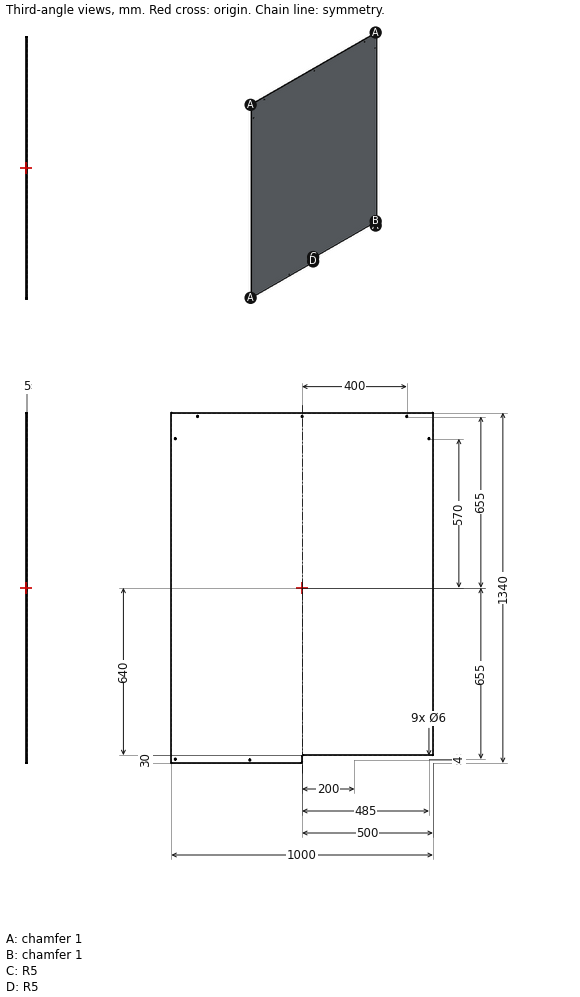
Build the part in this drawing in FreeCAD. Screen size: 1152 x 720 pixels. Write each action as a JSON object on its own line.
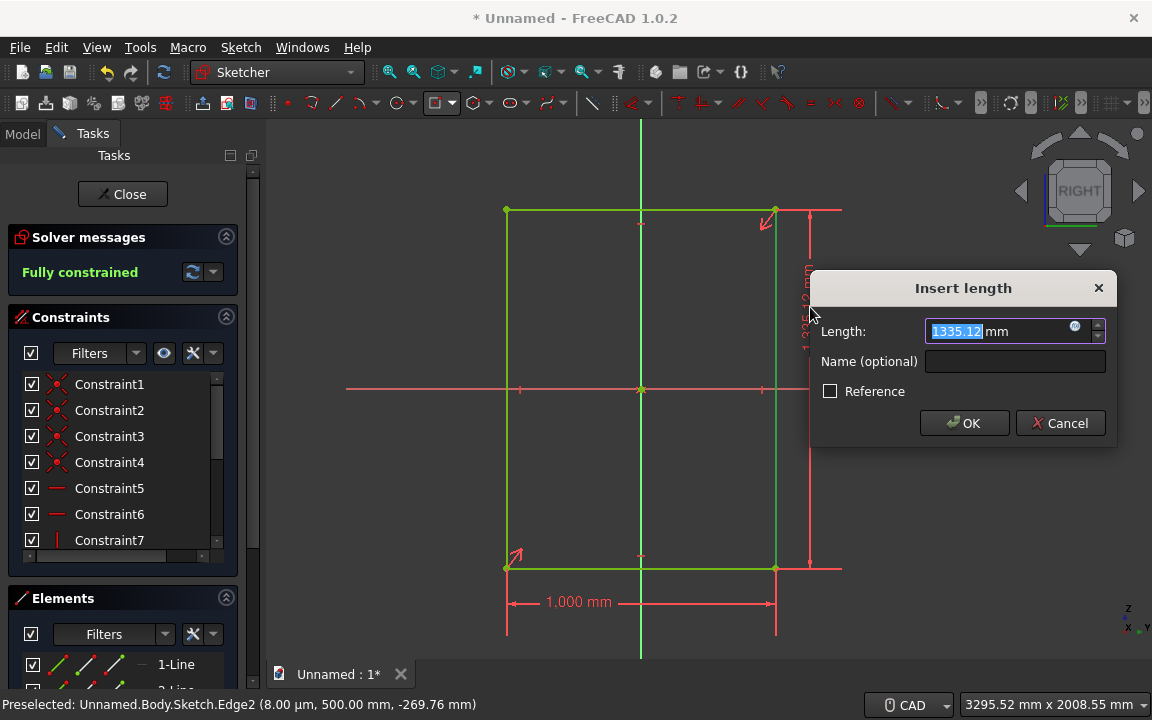
{"action": "type", "text": "1340"}
{"action": "key", "text": "Return"}
{"action": "key", "text": "Escape"}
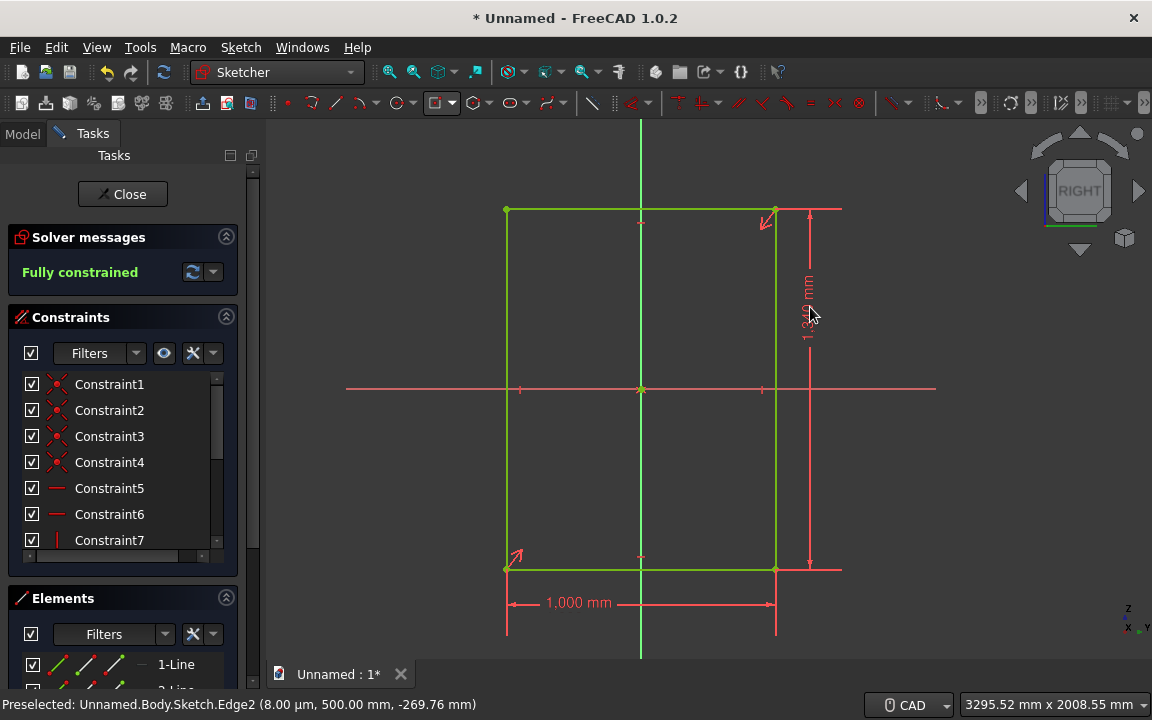
{"action": "left_click", "coordinate": [123, 194]}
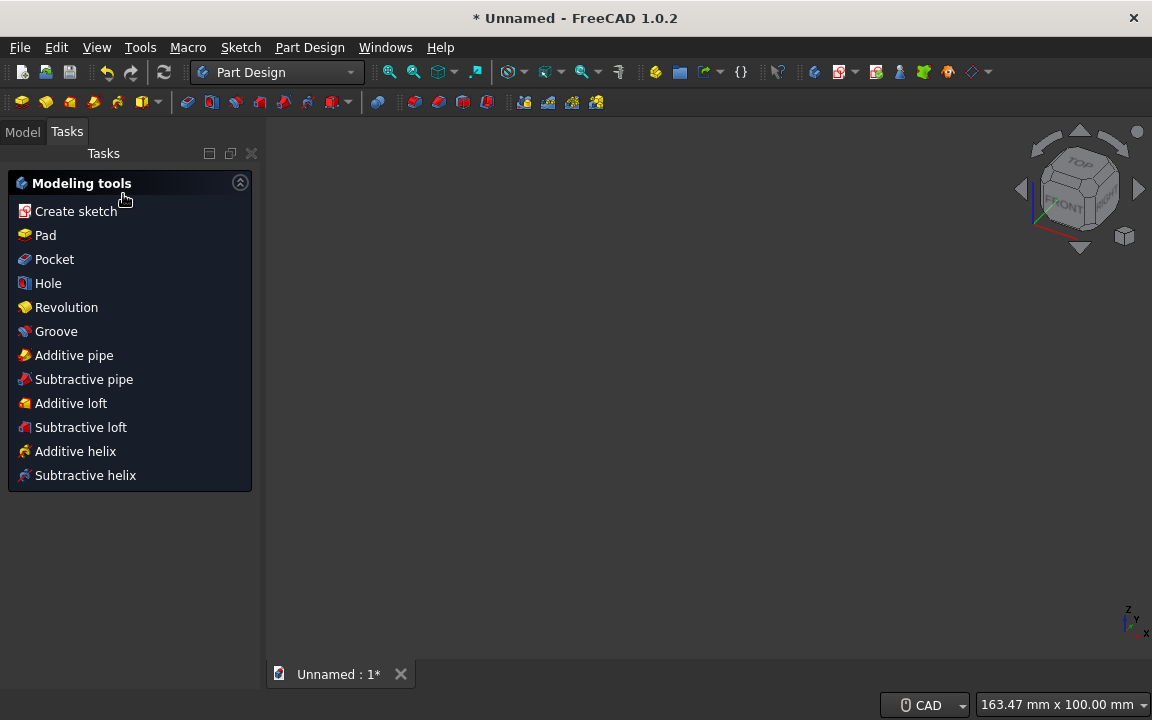
{"action": "left_click", "coordinate": [22, 102]}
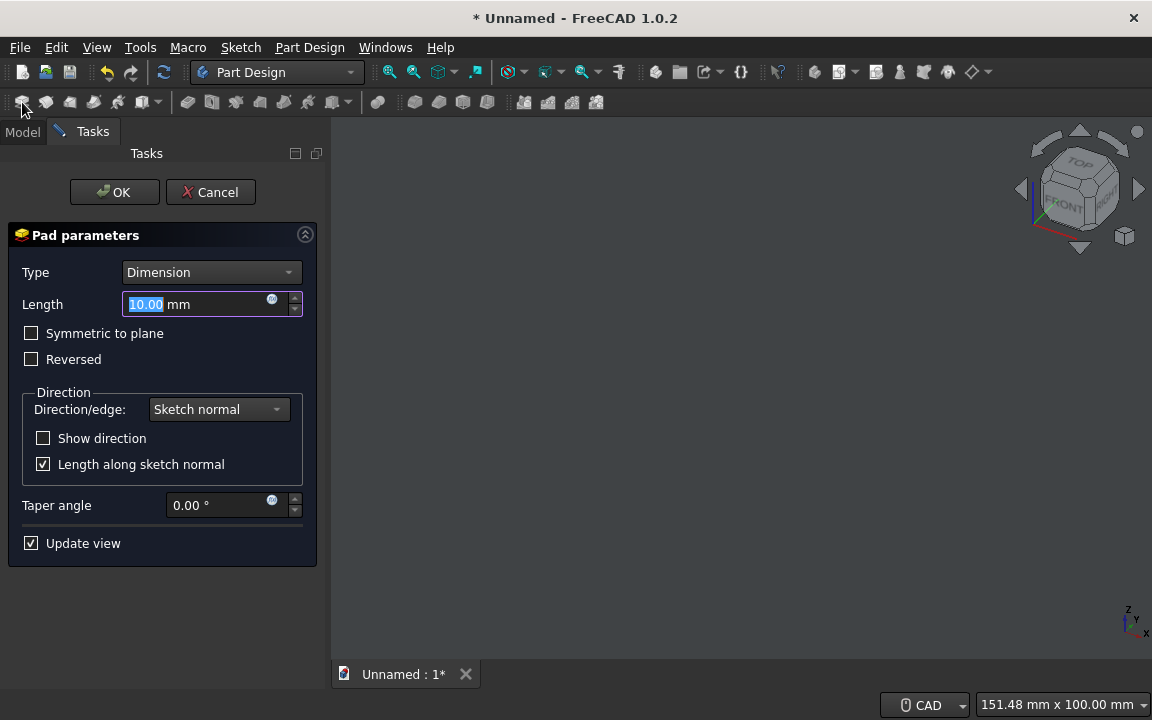
{"action": "type", "text": "5"}
{"action": "key", "text": "Tab"}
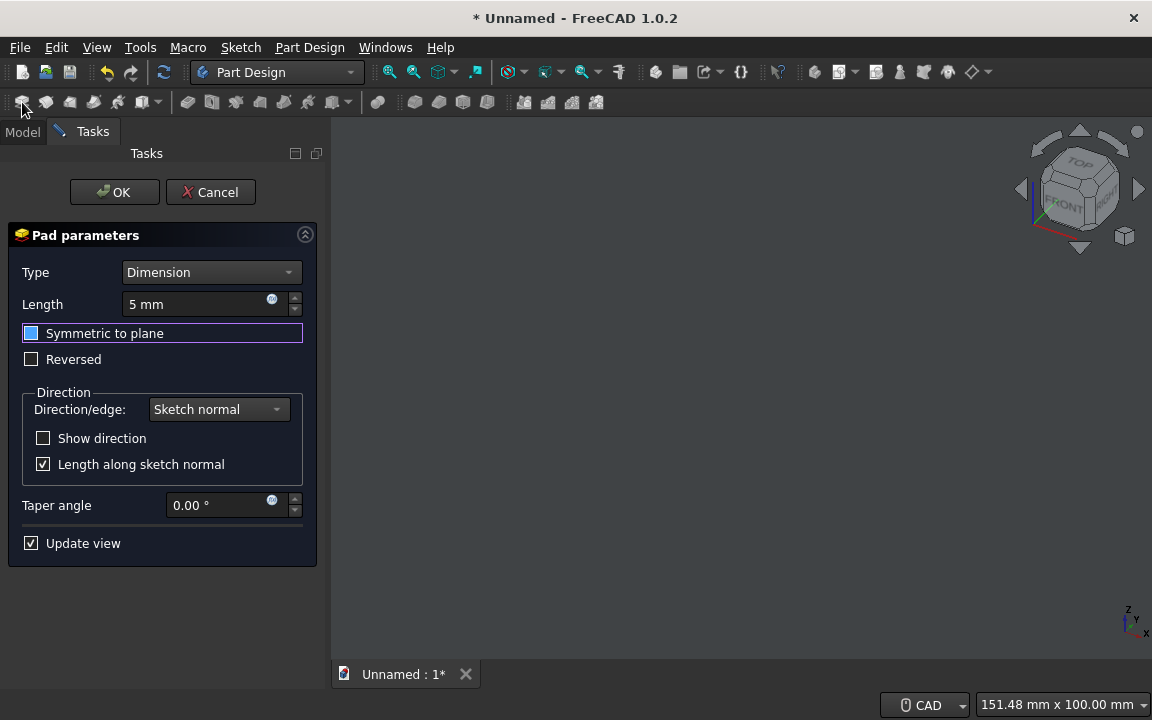
{"action": "left_click", "coordinate": [115, 192]}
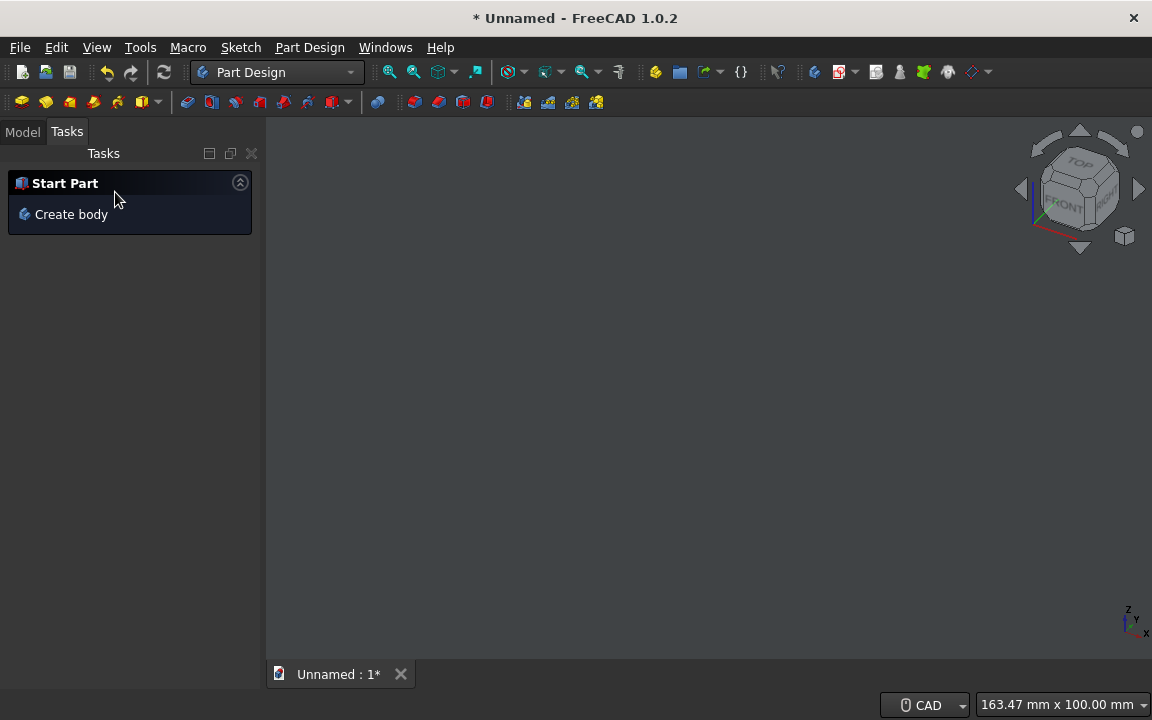
{"action": "left_click", "coordinate": [390, 72]}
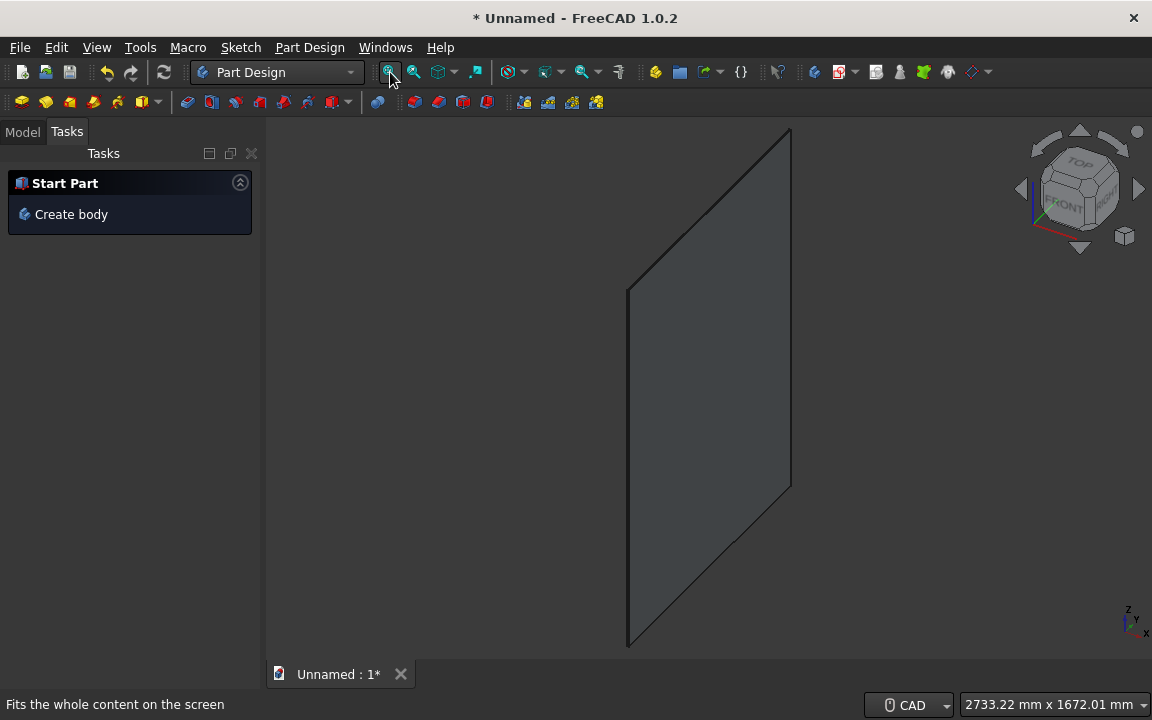
{"action": "key", "text": "0"}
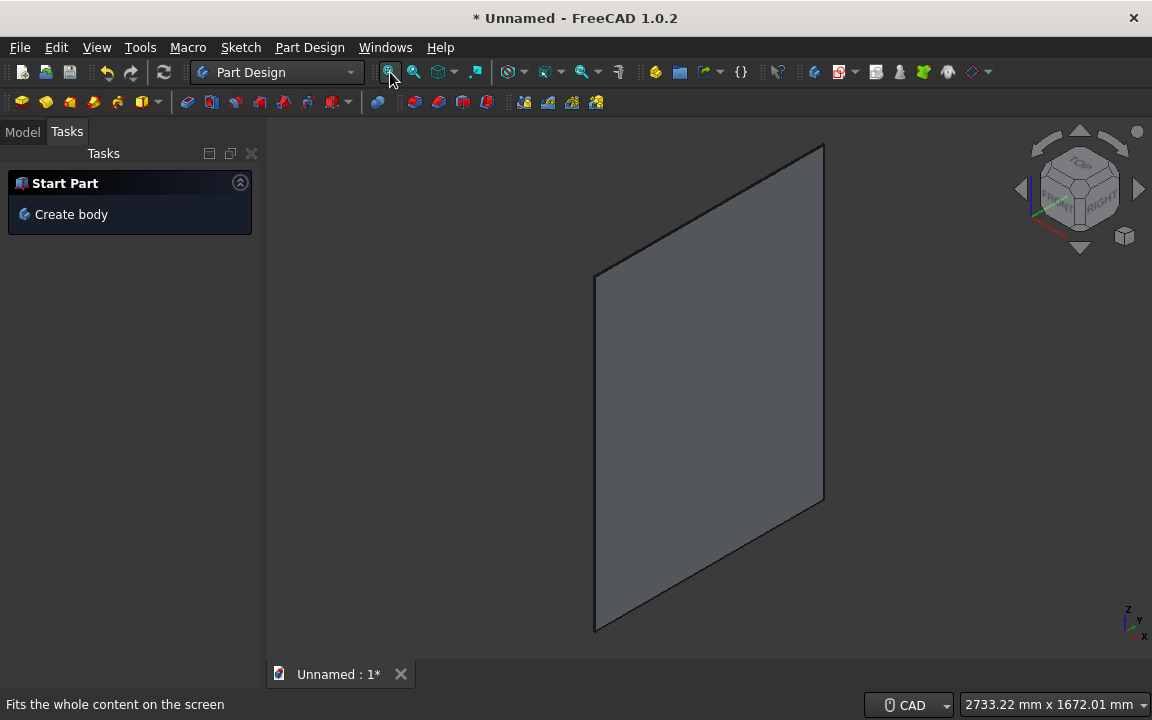
{"action": "key", "text": "2"}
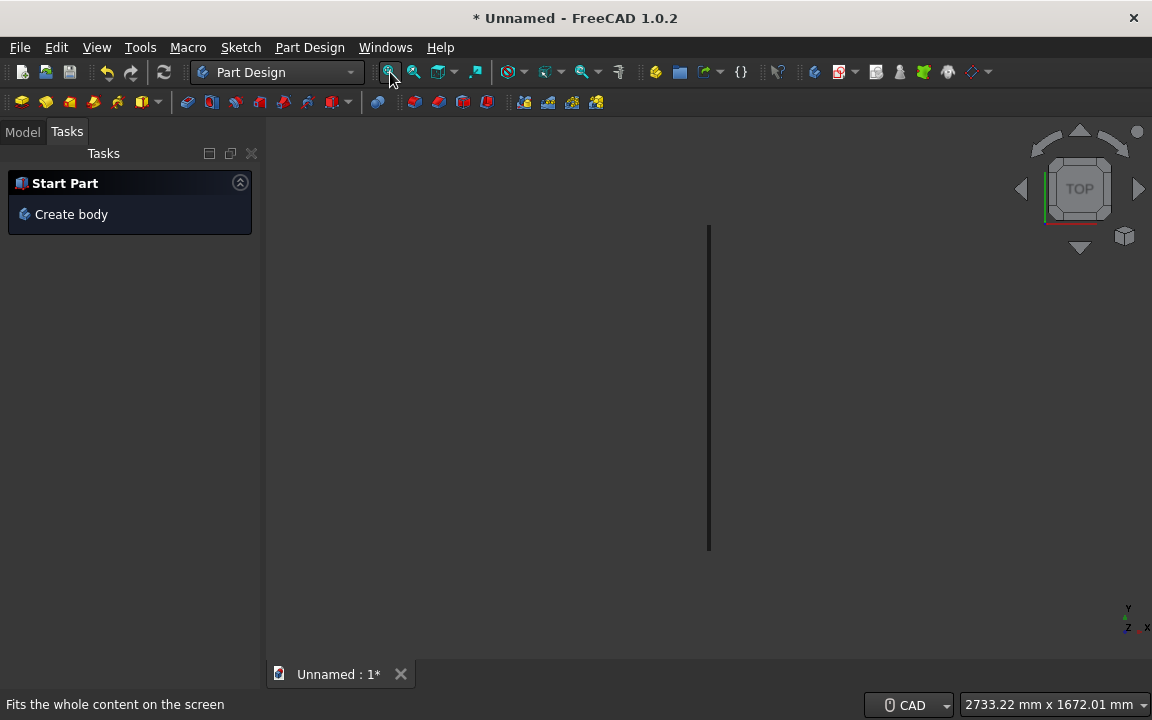
{"action": "scroll", "coordinate": [709, 225], "scroll_direction": "up", "scroll_amount": 15}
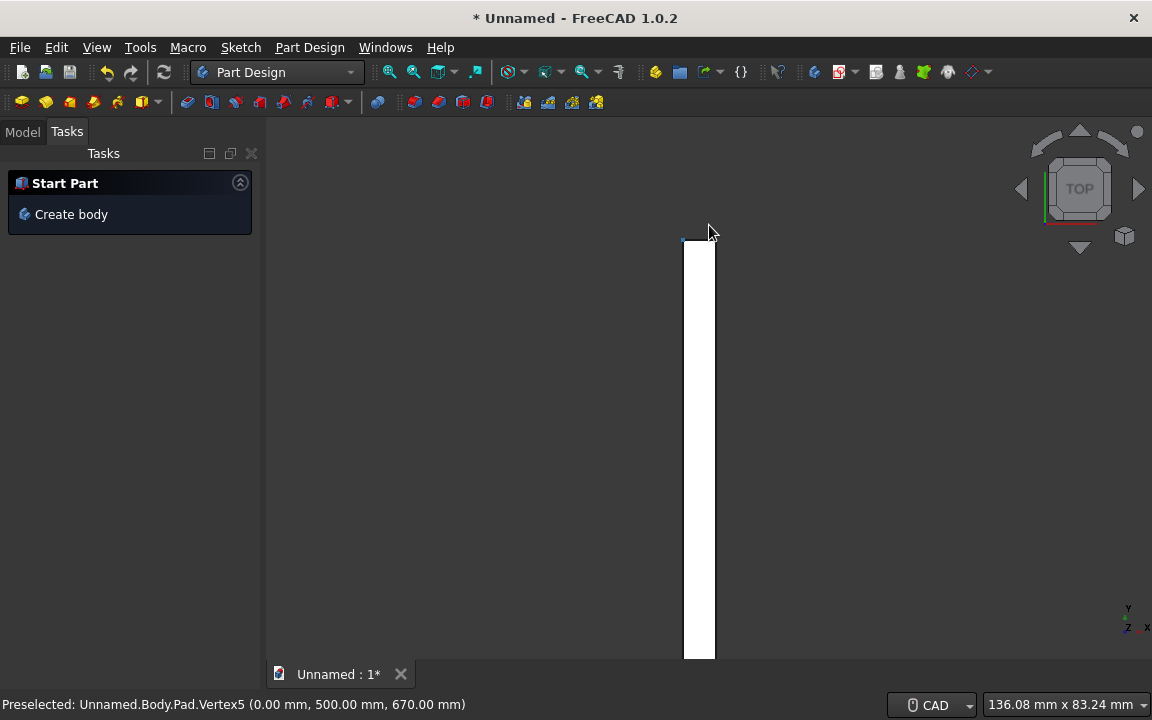
{"action": "left_click", "coordinate": [699, 239]}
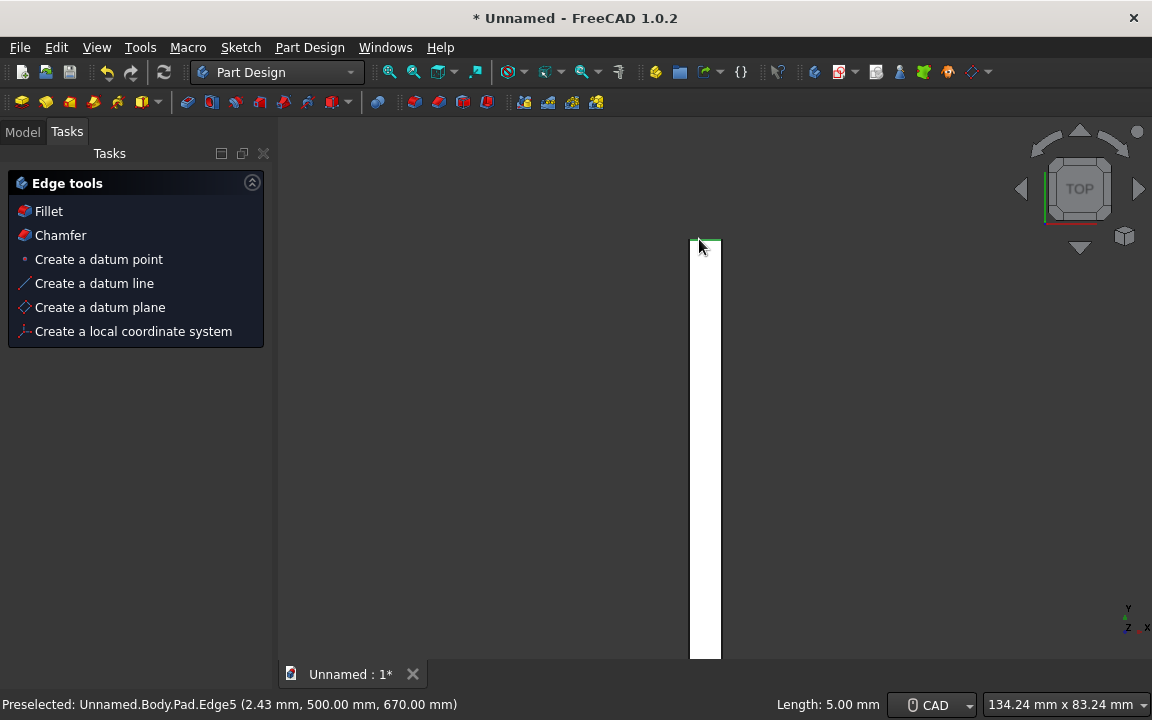
{"action": "left_click", "coordinate": [390, 72]}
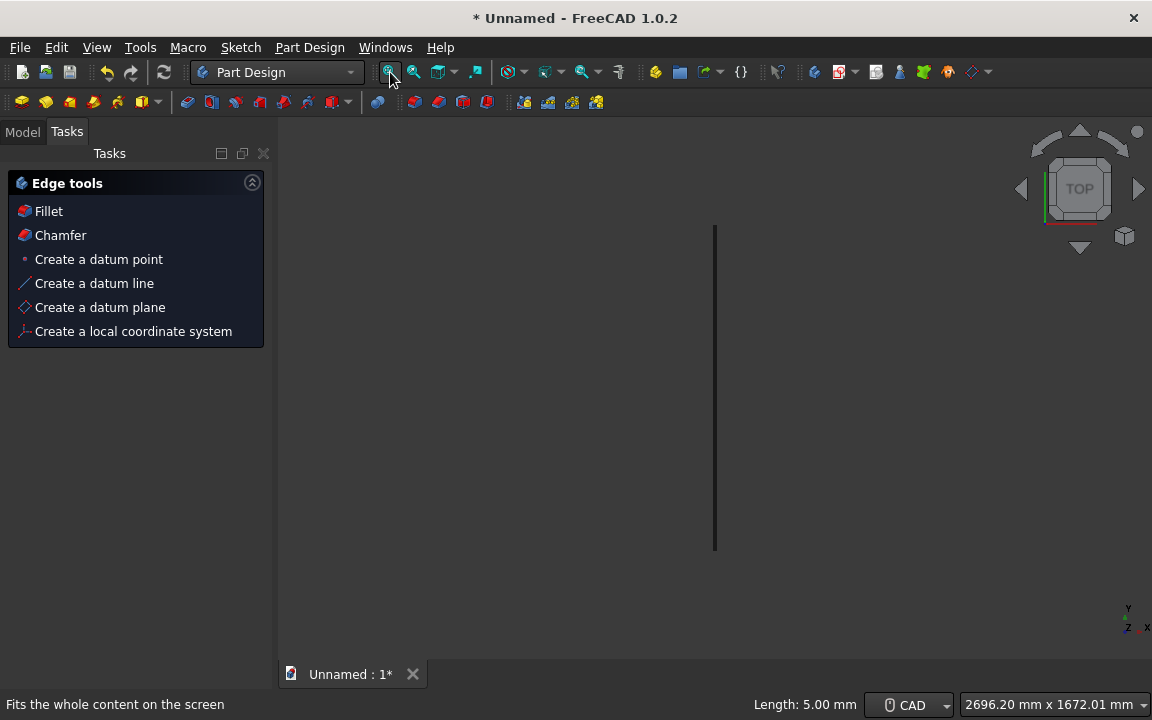
{"action": "key", "text": "1"}